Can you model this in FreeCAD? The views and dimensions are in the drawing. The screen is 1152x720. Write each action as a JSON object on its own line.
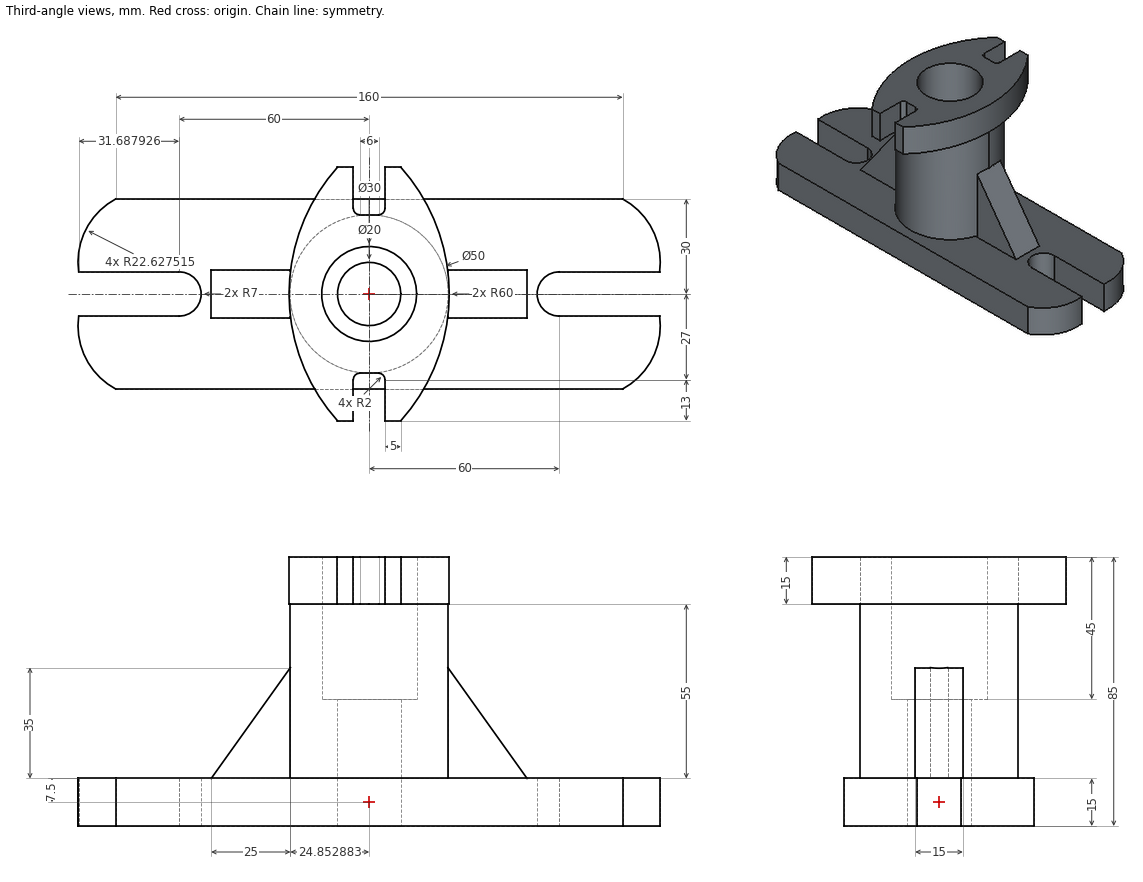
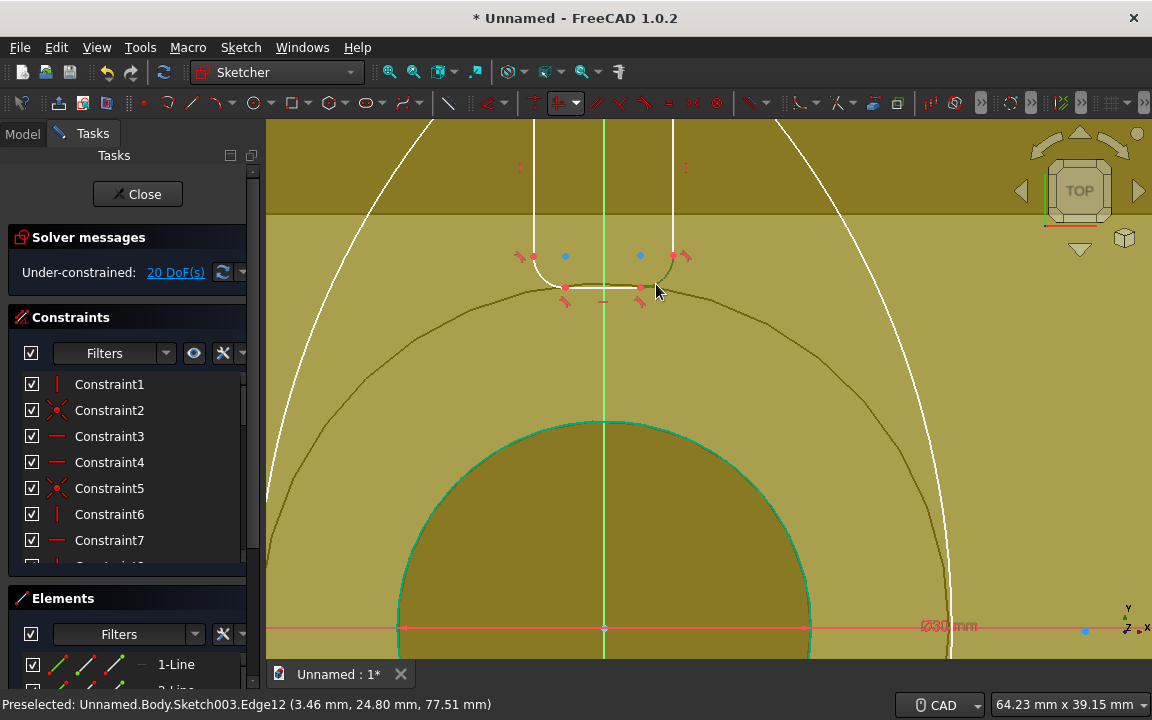
{"action": "left_click", "coordinate": [537, 271]}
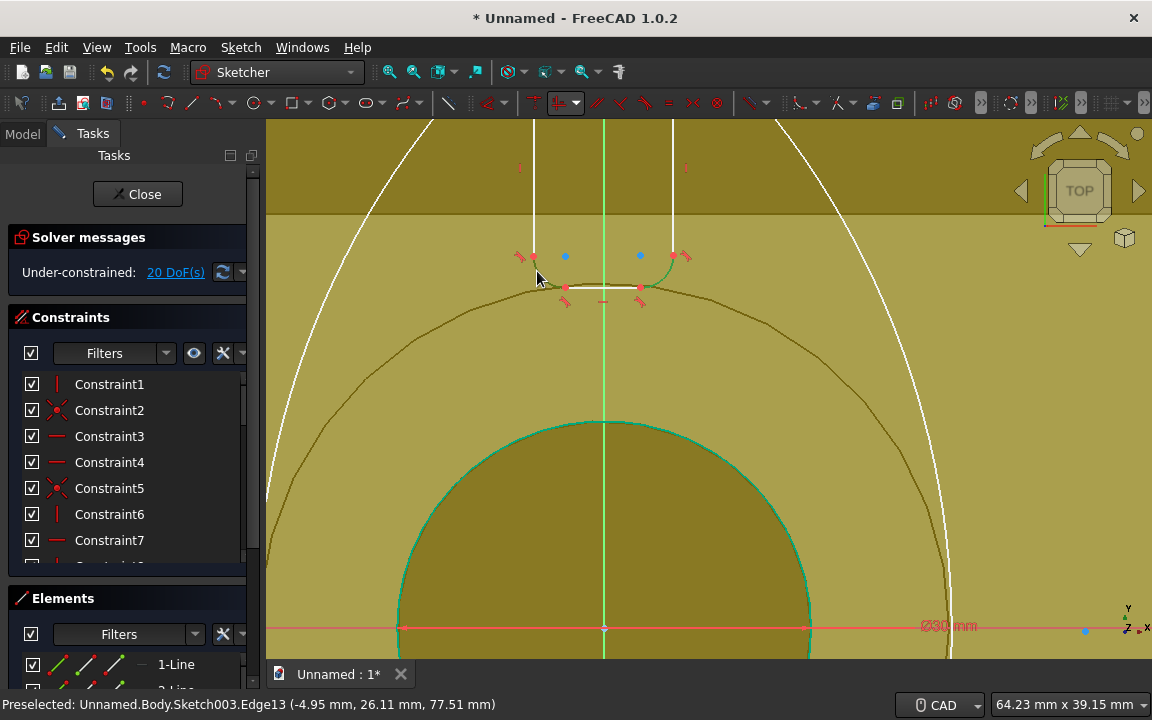
{"action": "scroll", "coordinate": [656, 286], "scroll_direction": "down", "scroll_amount": 6}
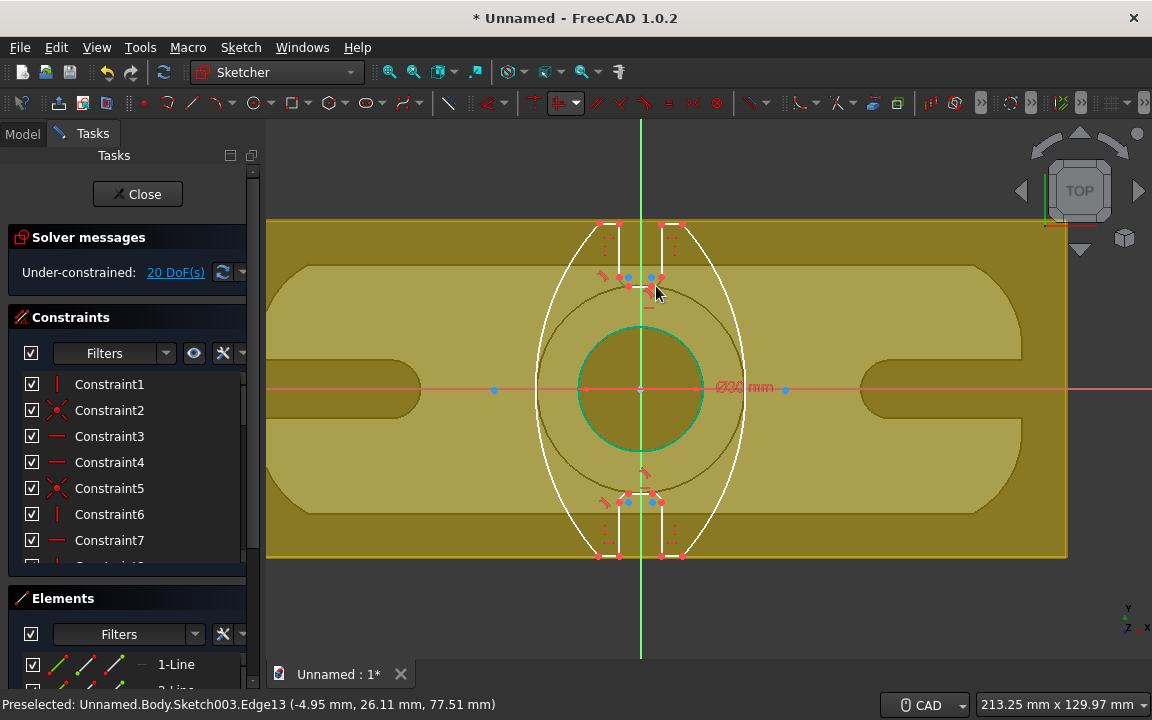
{"action": "scroll", "coordinate": [624, 494], "scroll_direction": "up", "scroll_amount": 7}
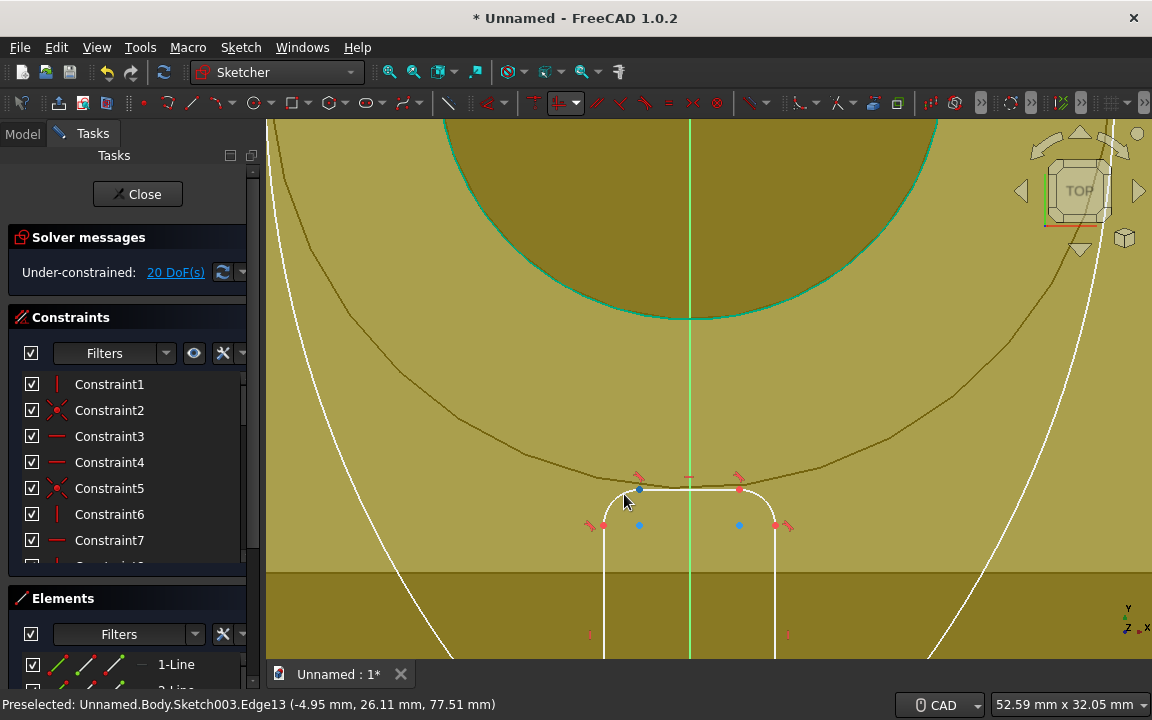
{"action": "left_click", "coordinate": [623, 494]}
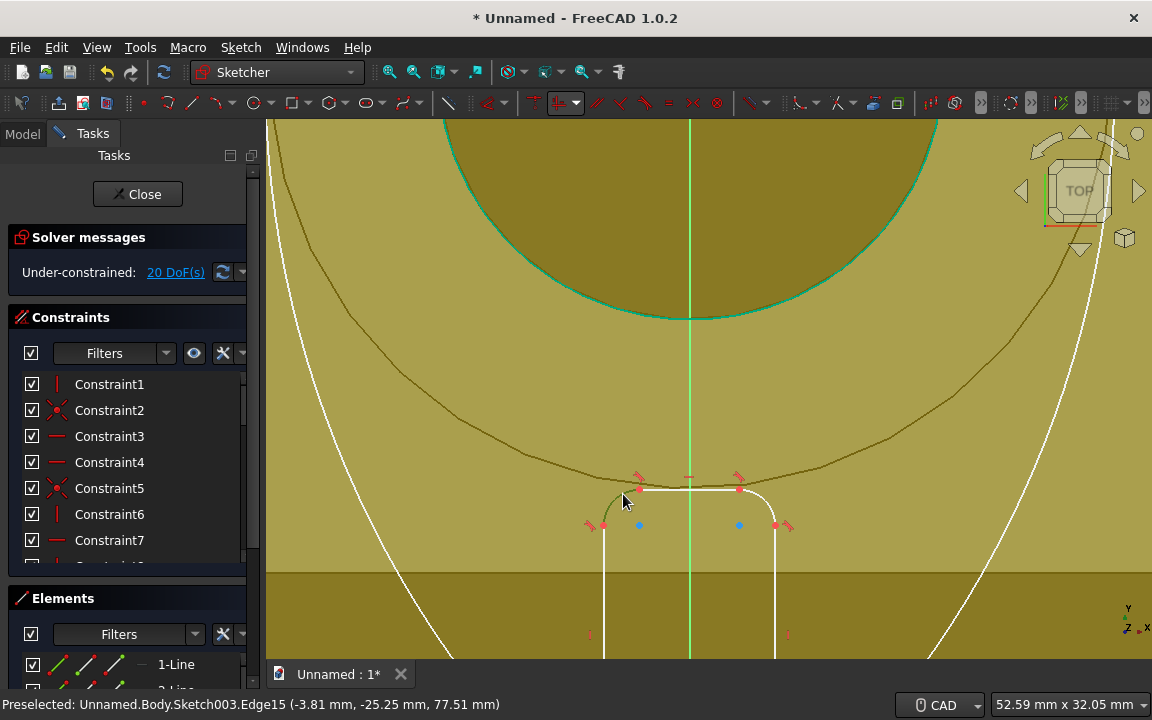
{"action": "left_click", "coordinate": [771, 509]}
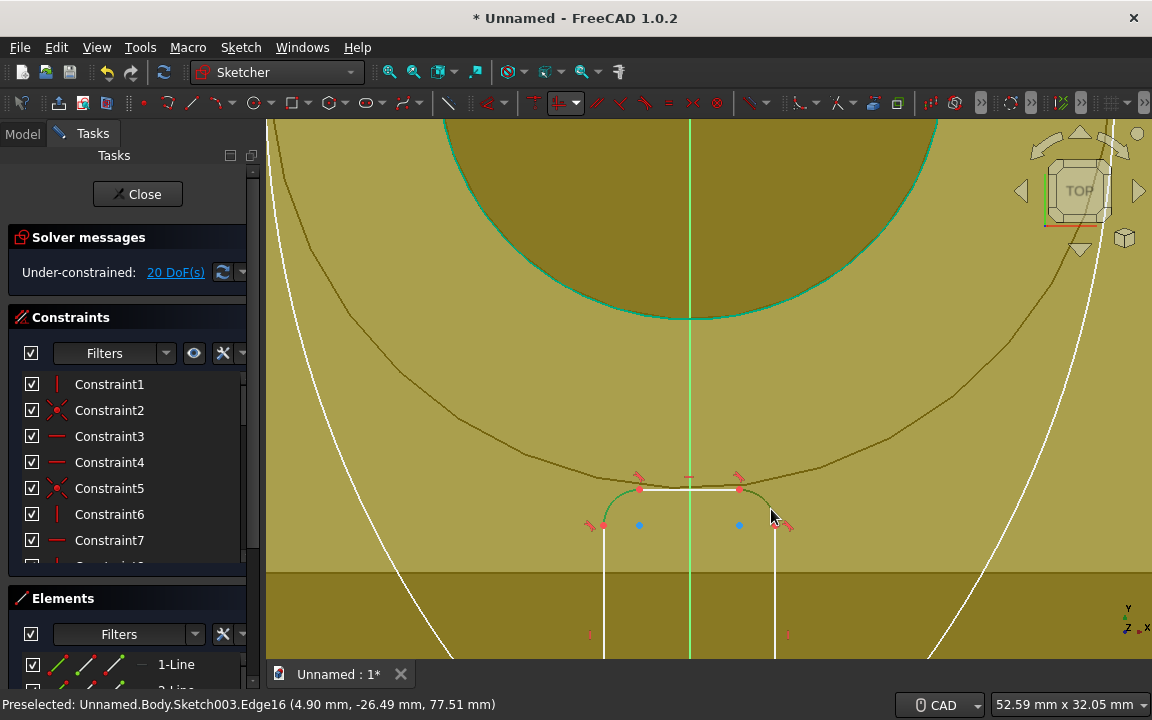
{"action": "key", "text": "e"}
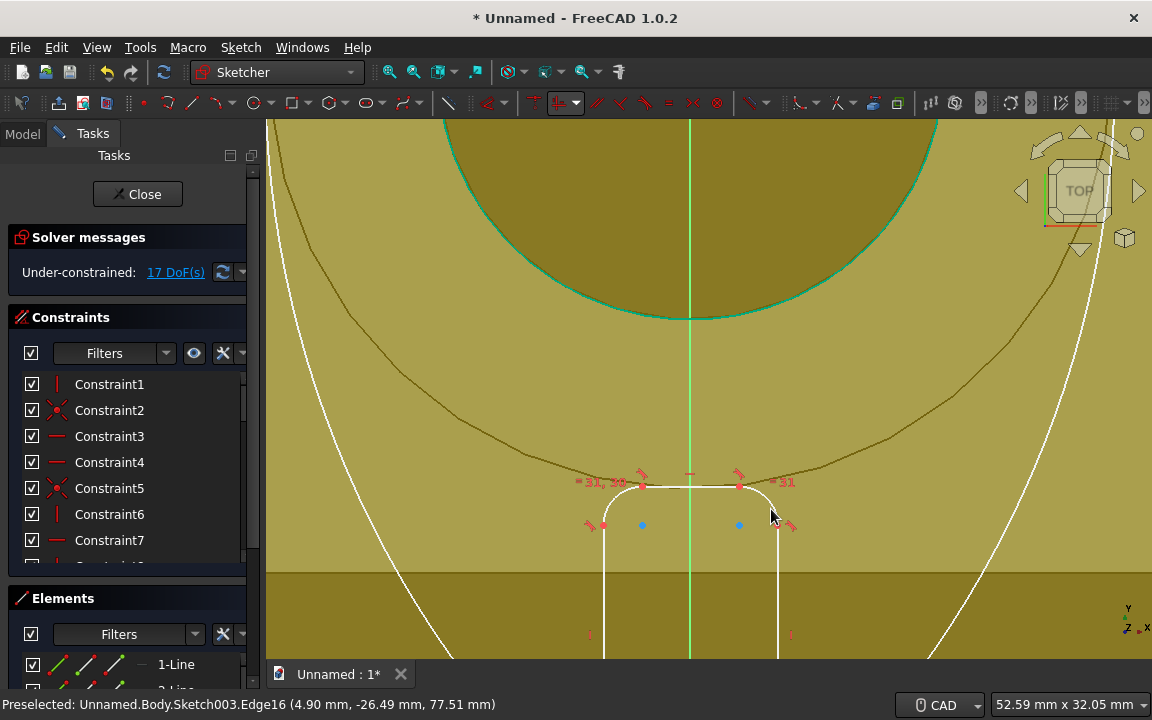
{"action": "scroll", "coordinate": [624, 494], "scroll_direction": "down", "scroll_amount": 7}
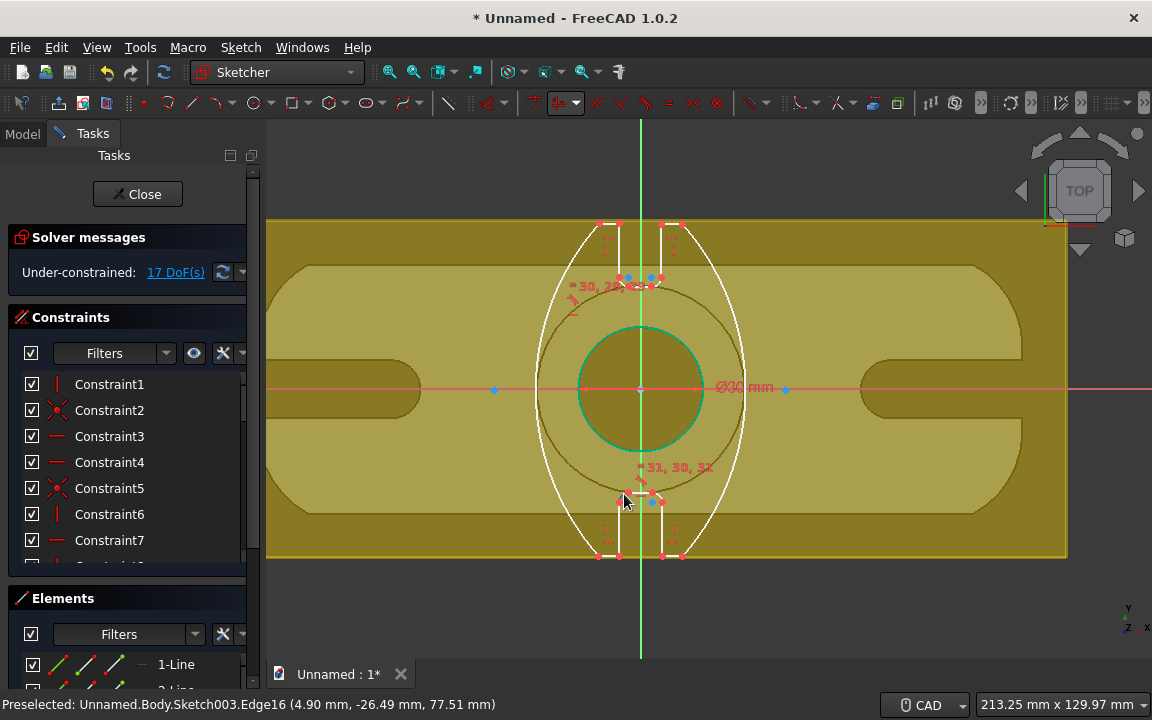
{"action": "left_click", "coordinate": [735, 462]}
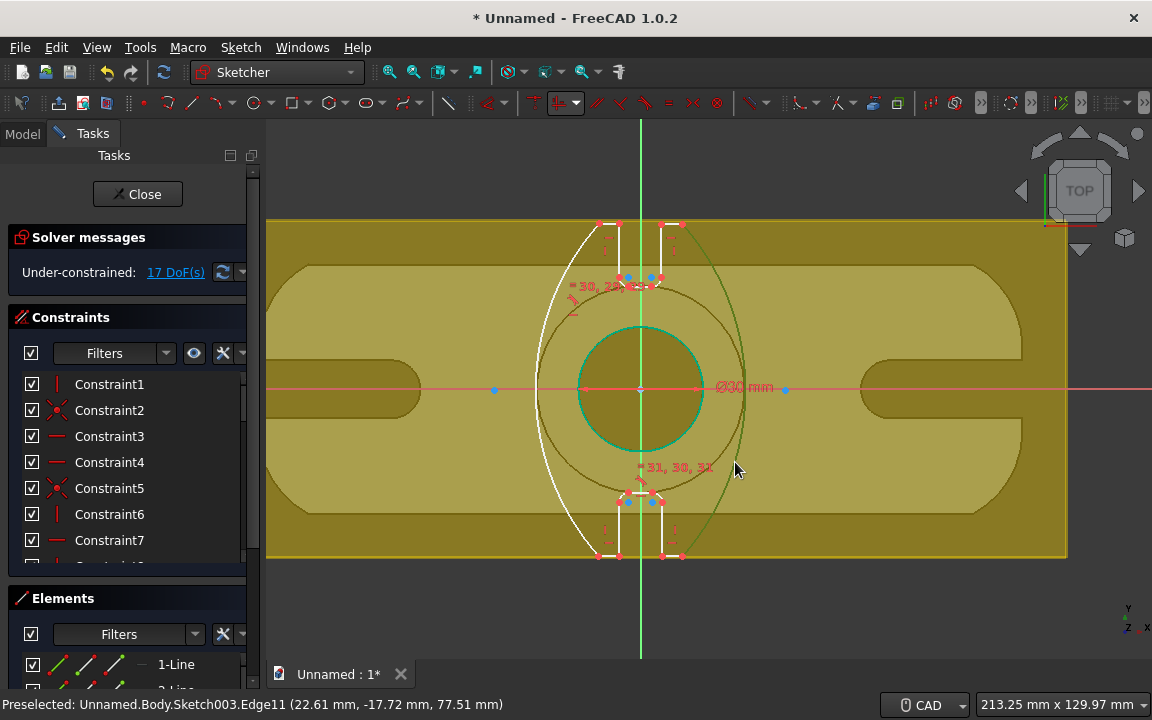
{"action": "left_click", "coordinate": [546, 318]}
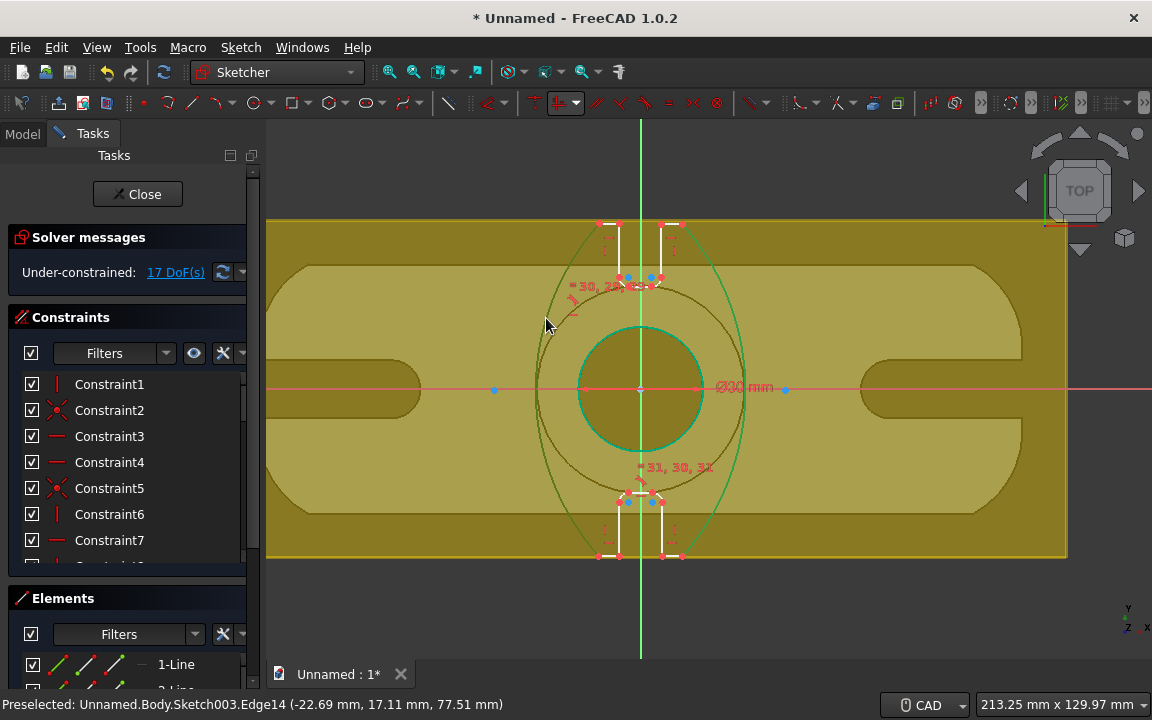
{"action": "key", "text": "e"}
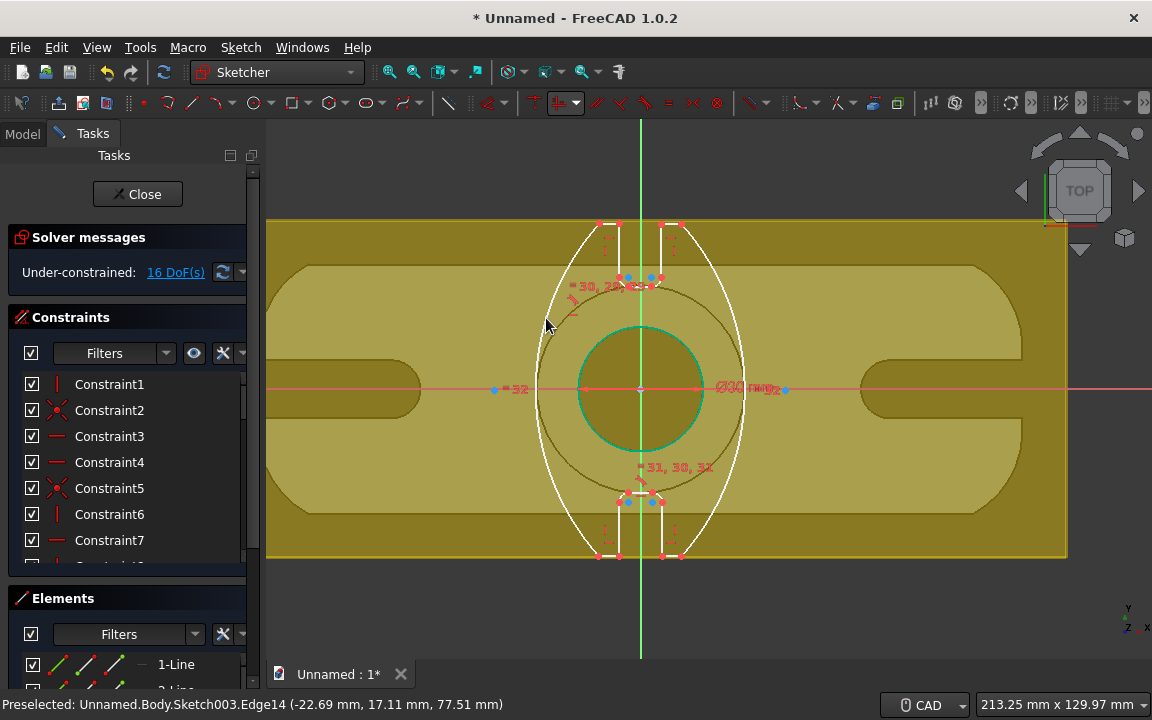
{"action": "left_click", "coordinate": [495, 390]}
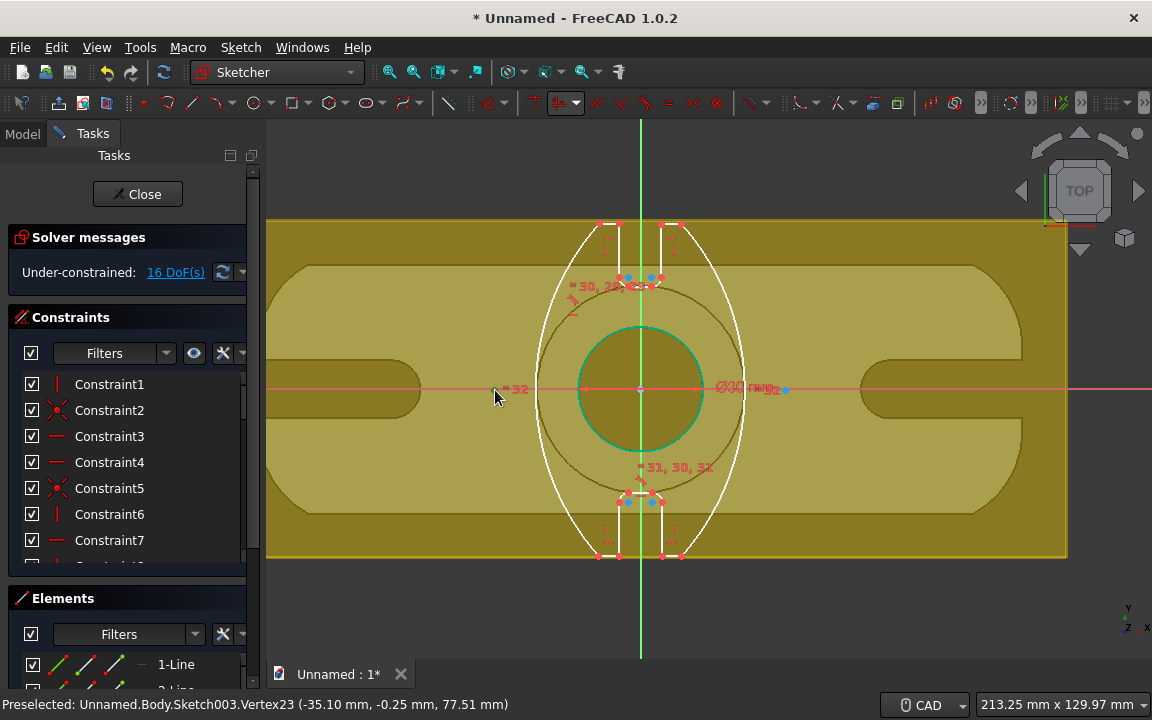
{"action": "left_click", "coordinate": [344, 389]}